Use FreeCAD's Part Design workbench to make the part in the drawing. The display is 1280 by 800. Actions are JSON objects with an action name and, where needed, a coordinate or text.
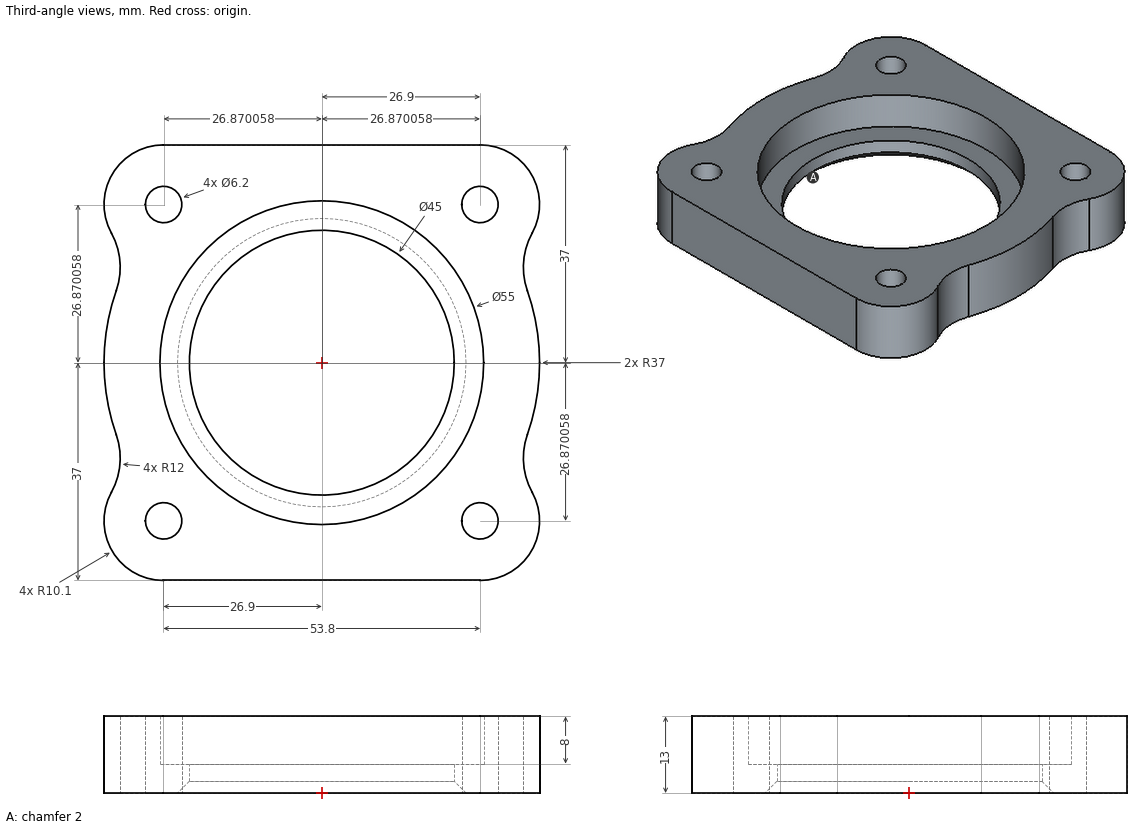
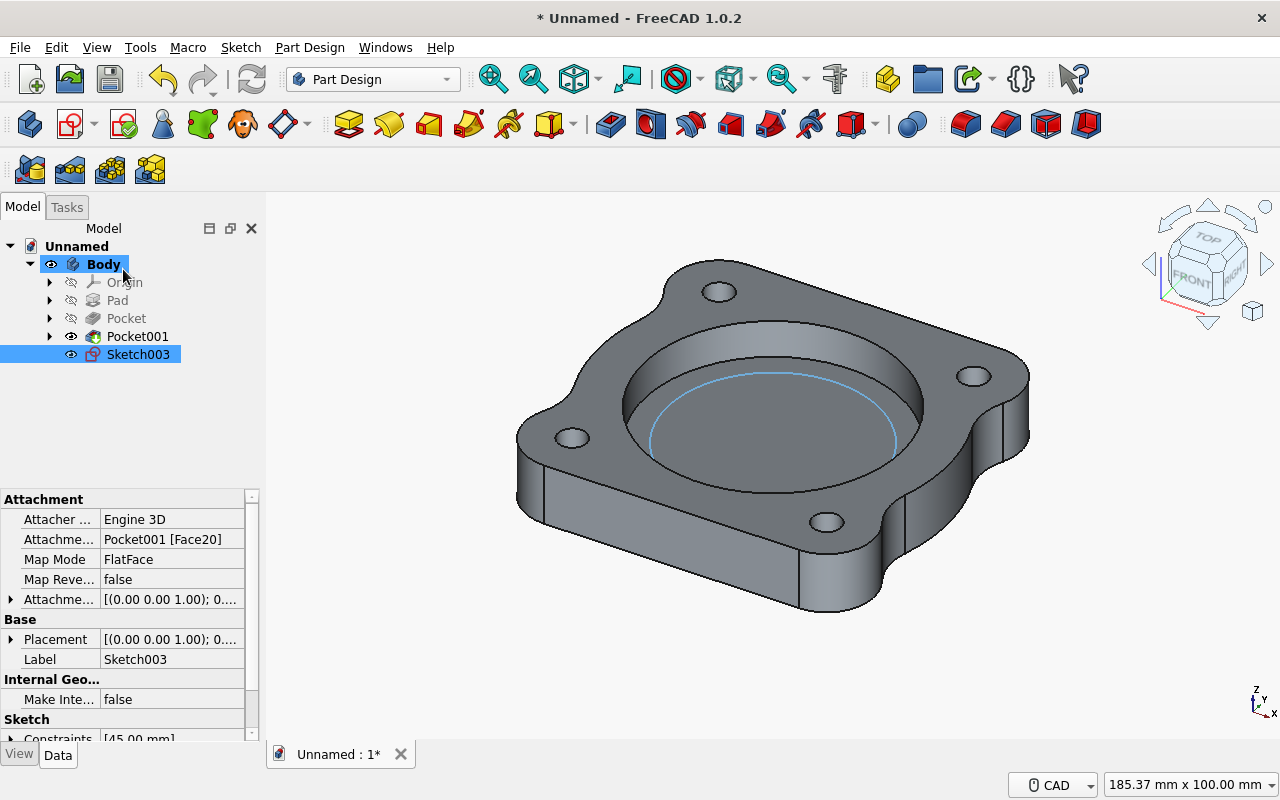
{"action": "left_click", "coordinate": [612, 124]}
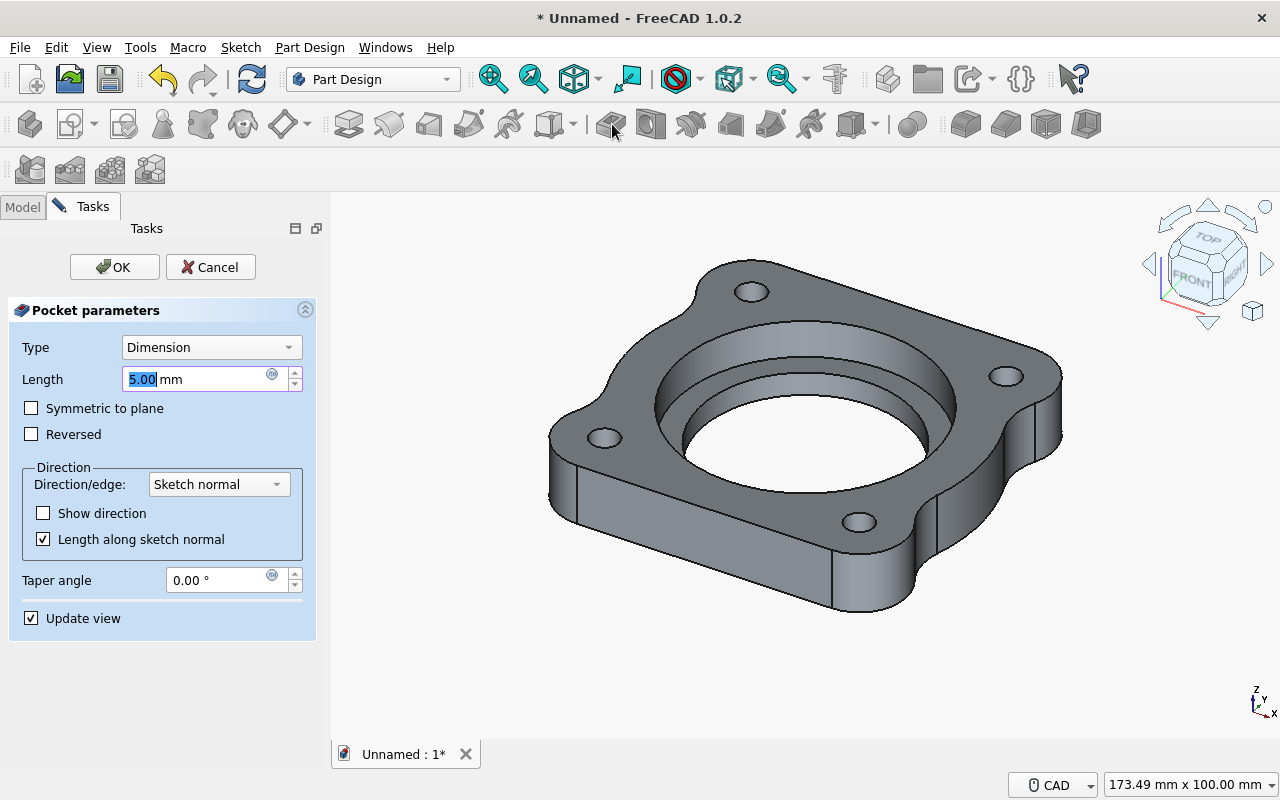
{"action": "left_click", "coordinate": [212, 348]}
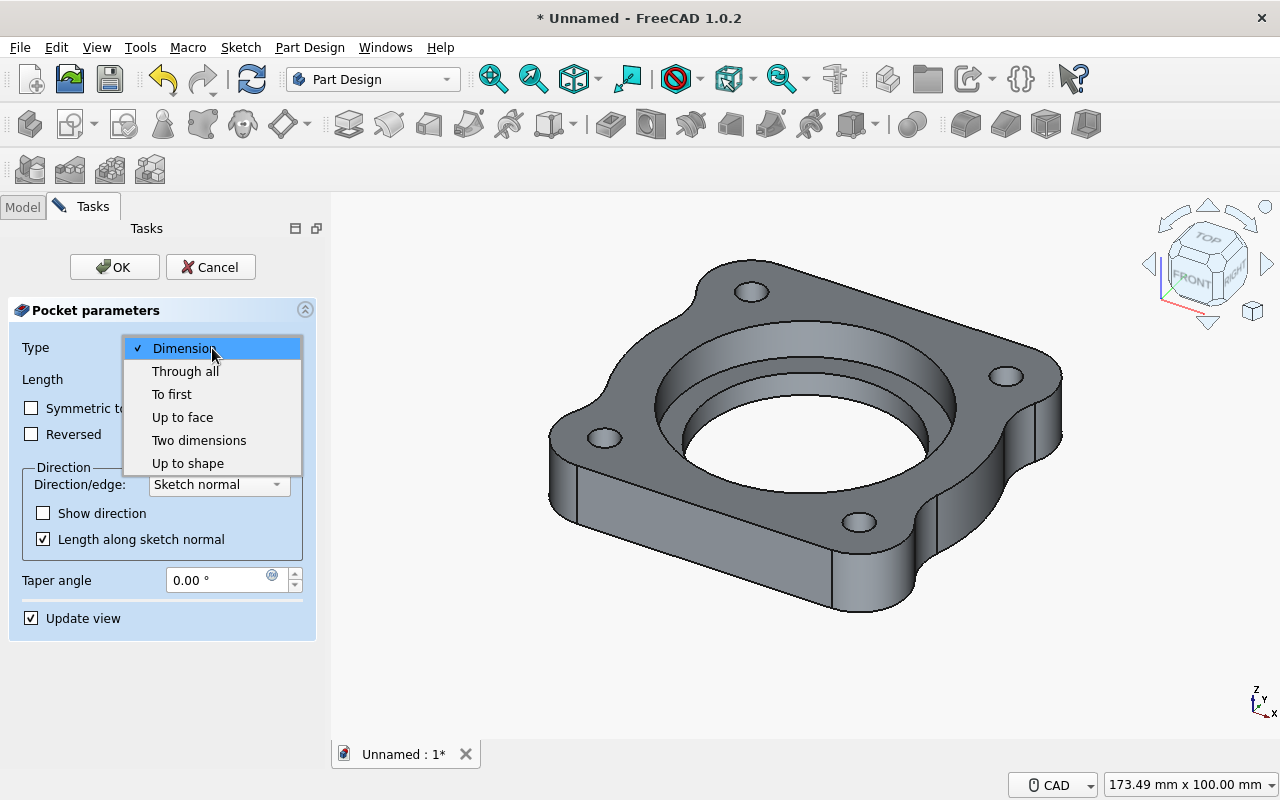
{"action": "left_click", "coordinate": [212, 394]}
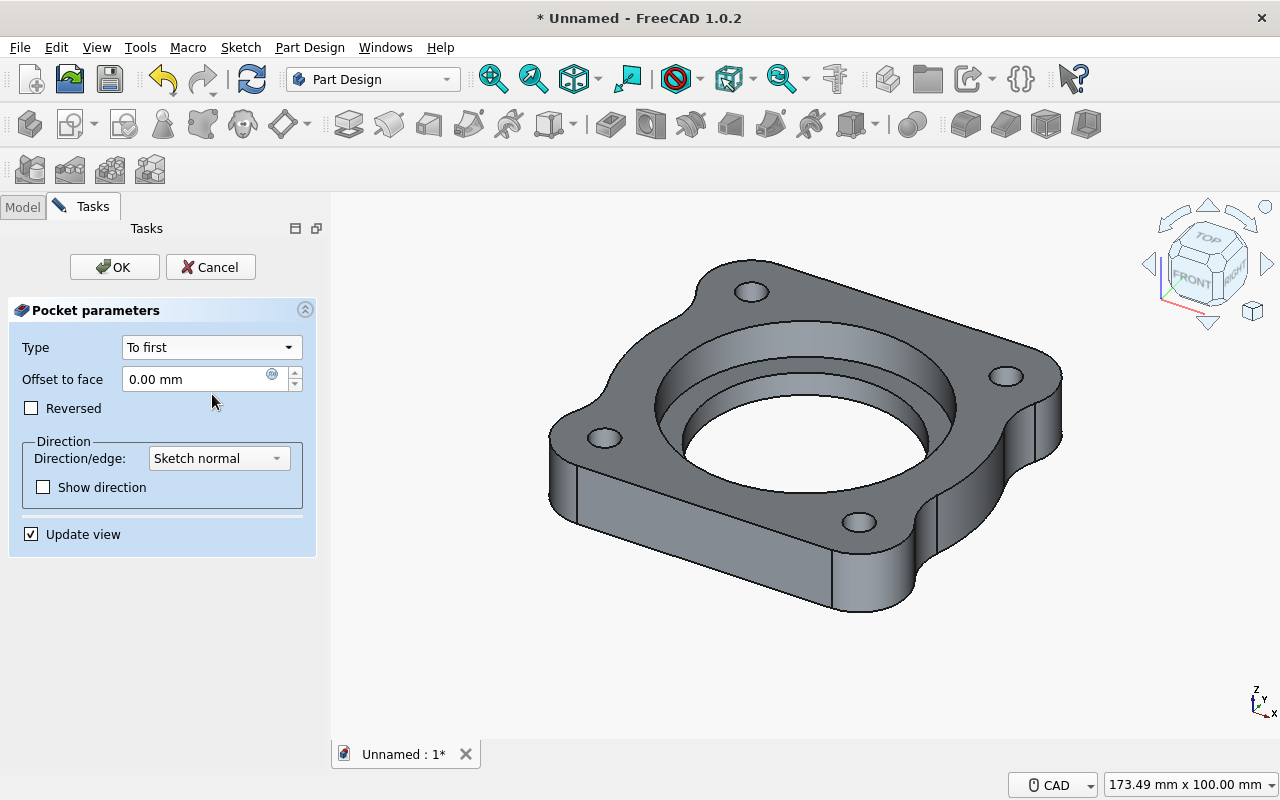
{"action": "left_click", "coordinate": [115, 267]}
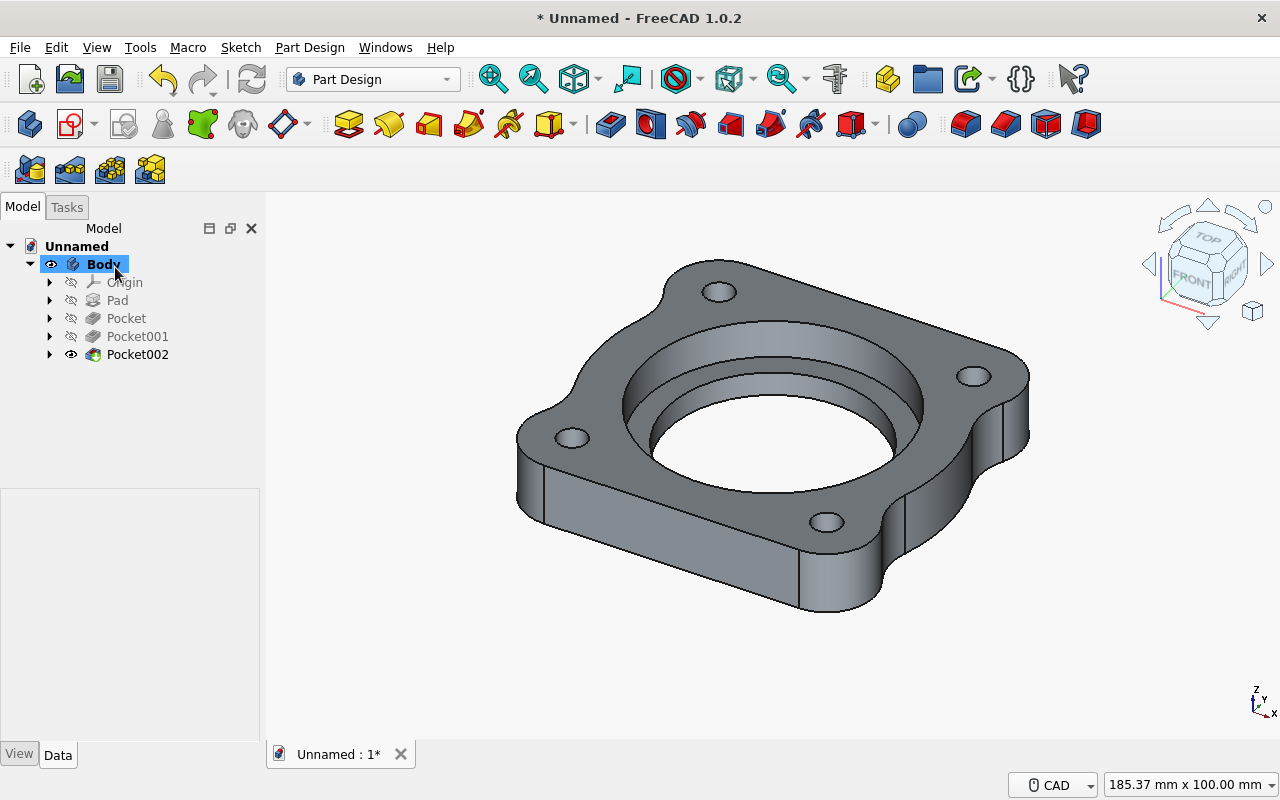
{"action": "key", "text": "0"}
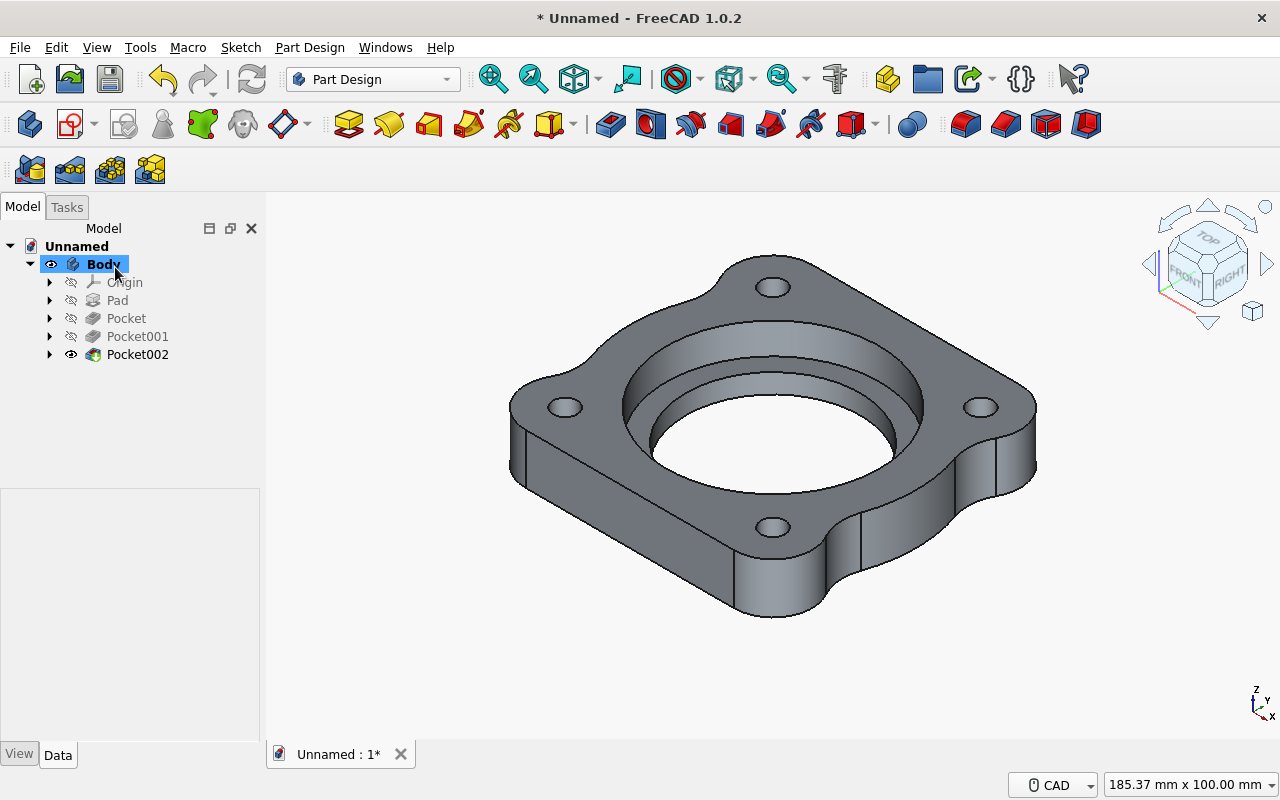
{"action": "key", "text": "2"}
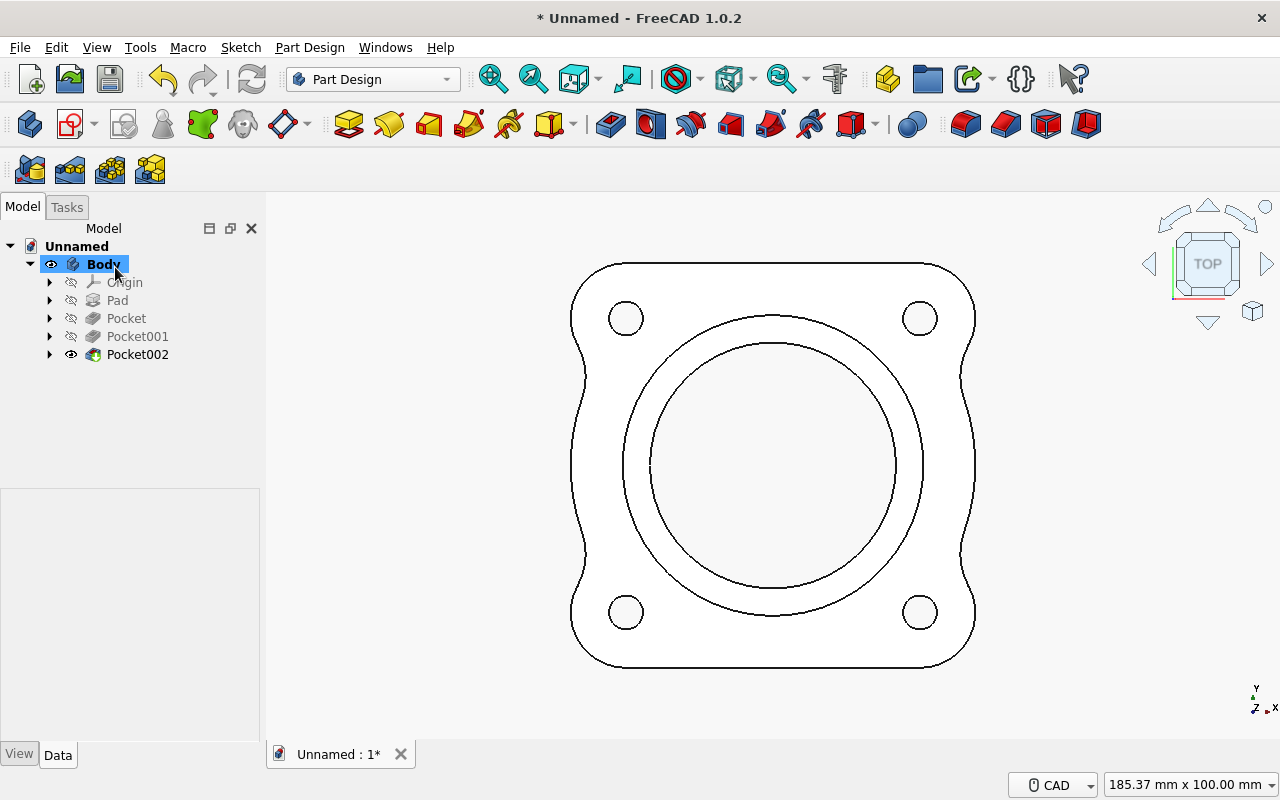
{"action": "key", "text": "1"}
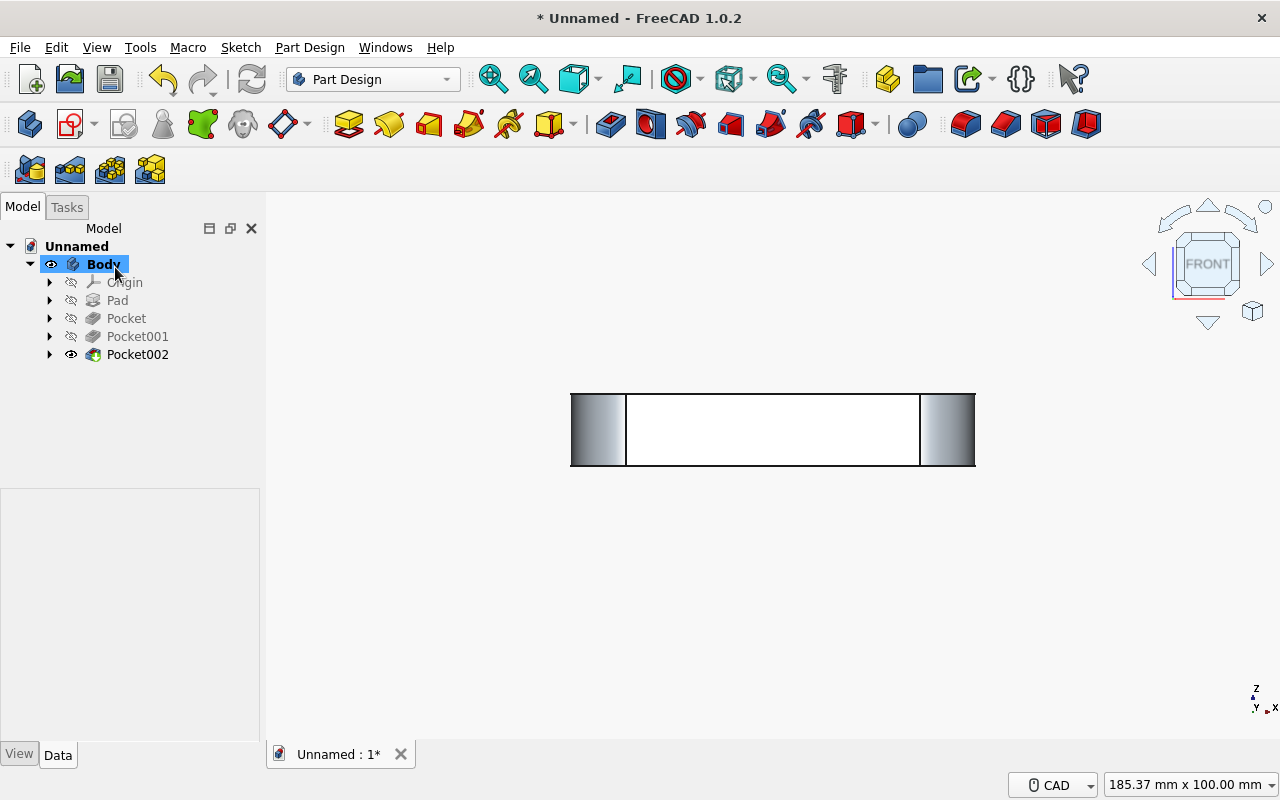
{"action": "left_click", "coordinate": [494, 80]}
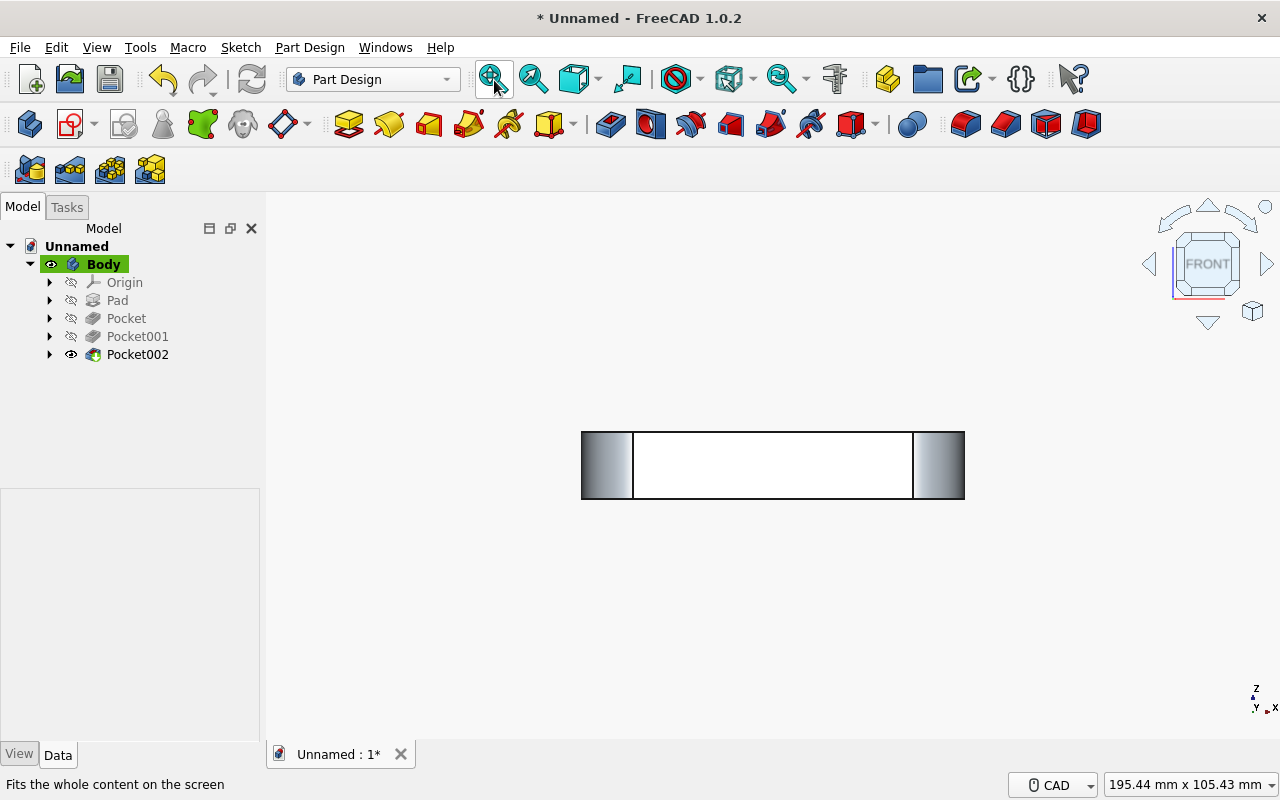
{"action": "key", "text": "3"}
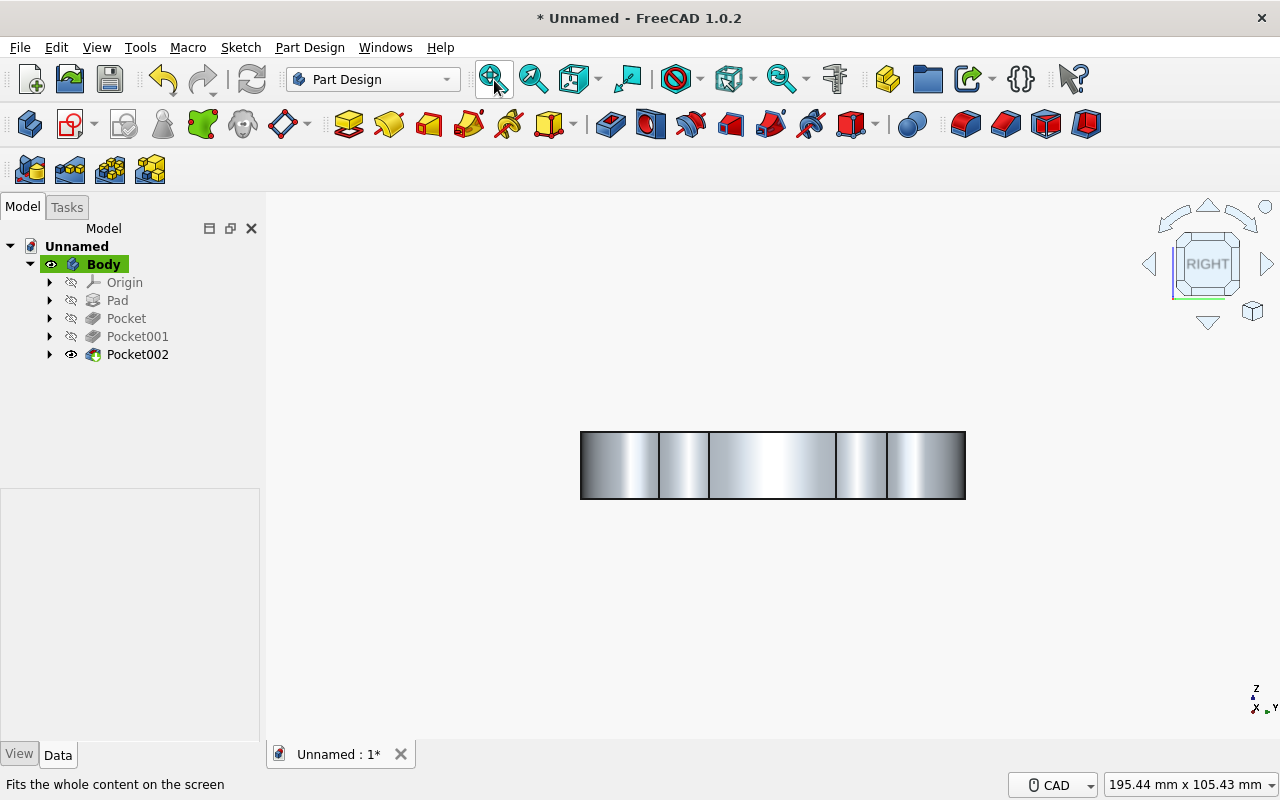
{"action": "left_click", "coordinate": [494, 80]}